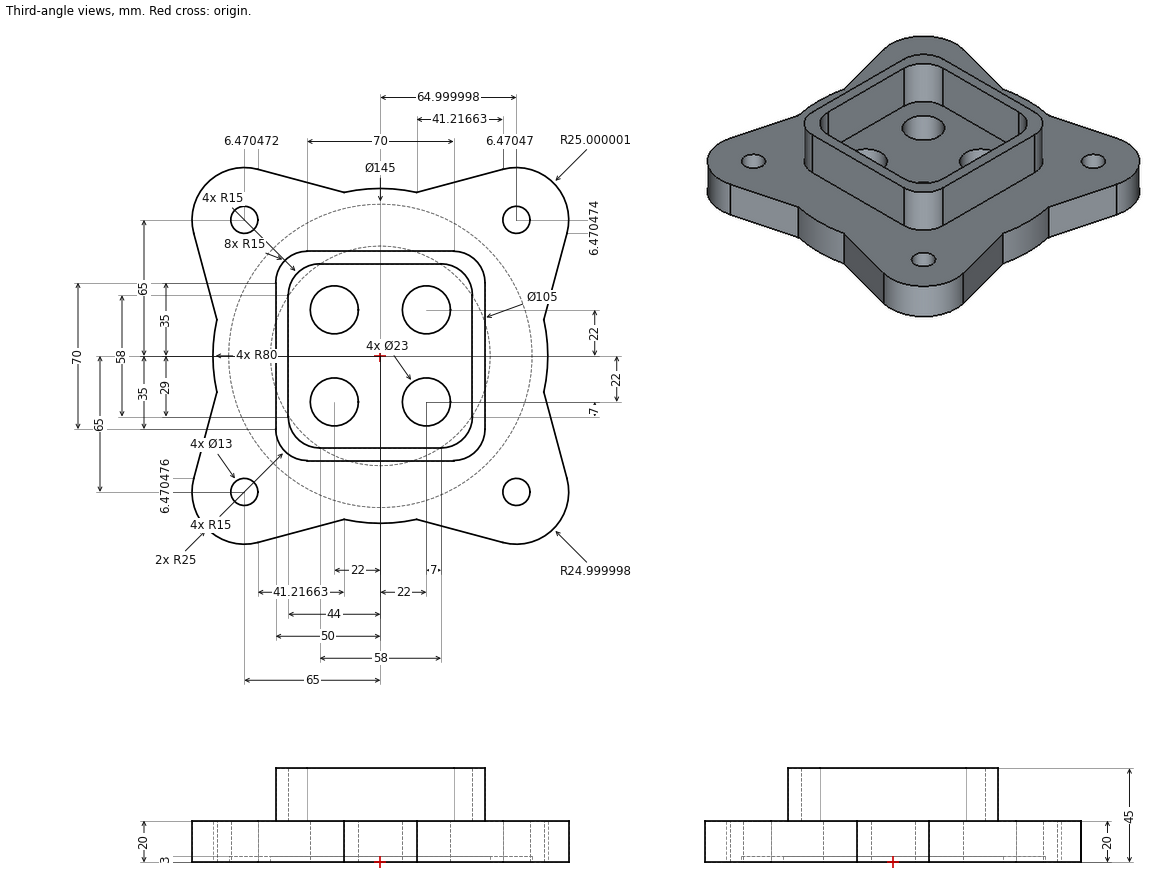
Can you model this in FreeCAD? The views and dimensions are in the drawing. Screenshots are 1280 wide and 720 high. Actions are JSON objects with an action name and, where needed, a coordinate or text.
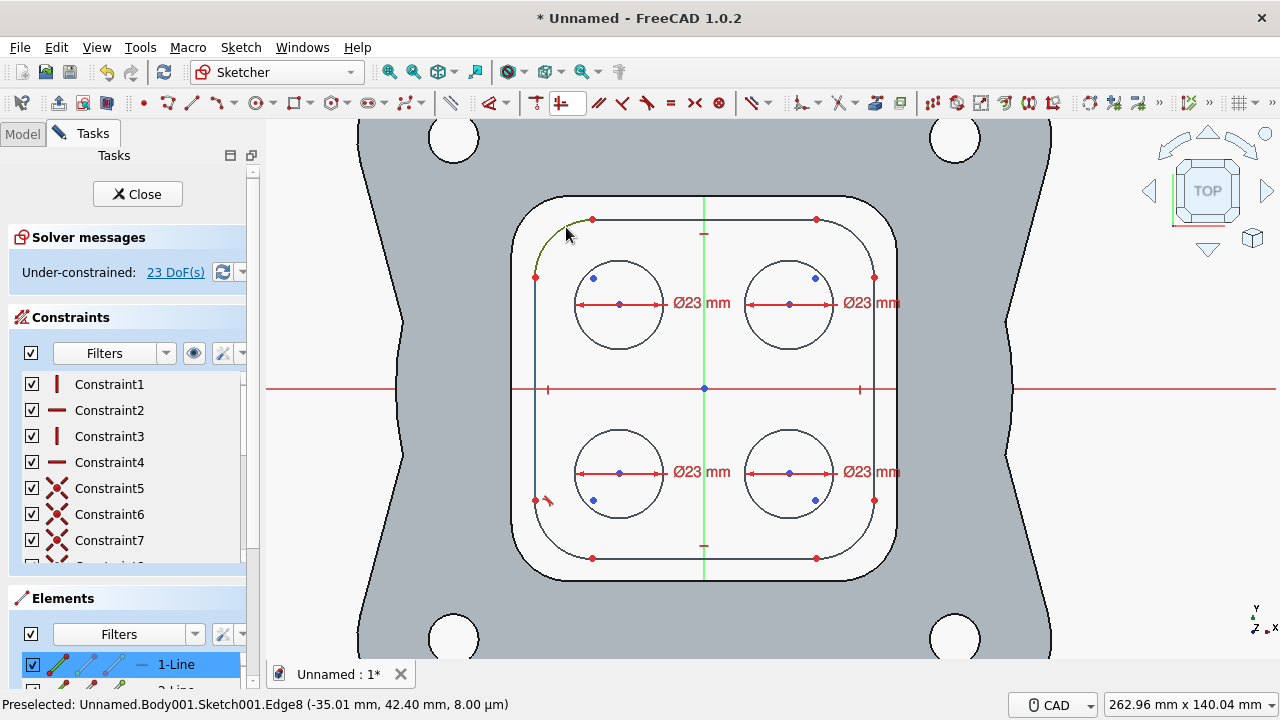
{"action": "left_click", "coordinate": [648, 104]}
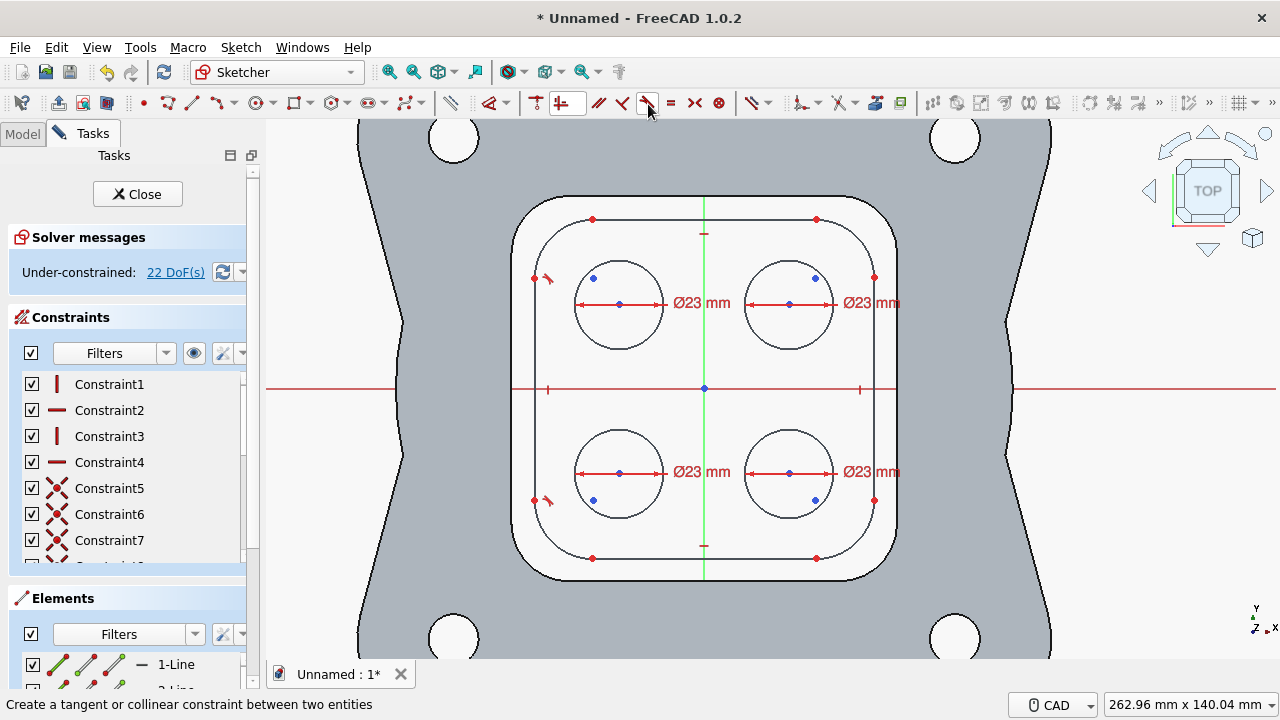
{"action": "left_click", "coordinate": [659, 559]}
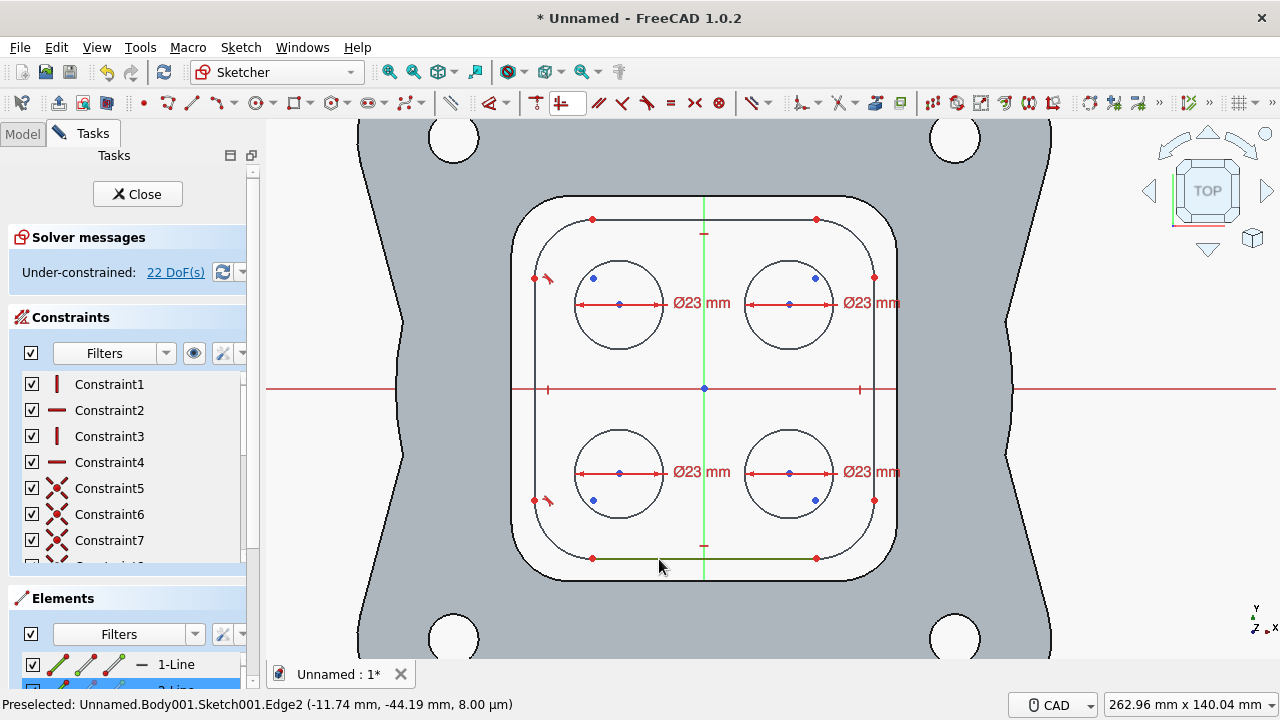
{"action": "left_click", "coordinate": [541, 527]}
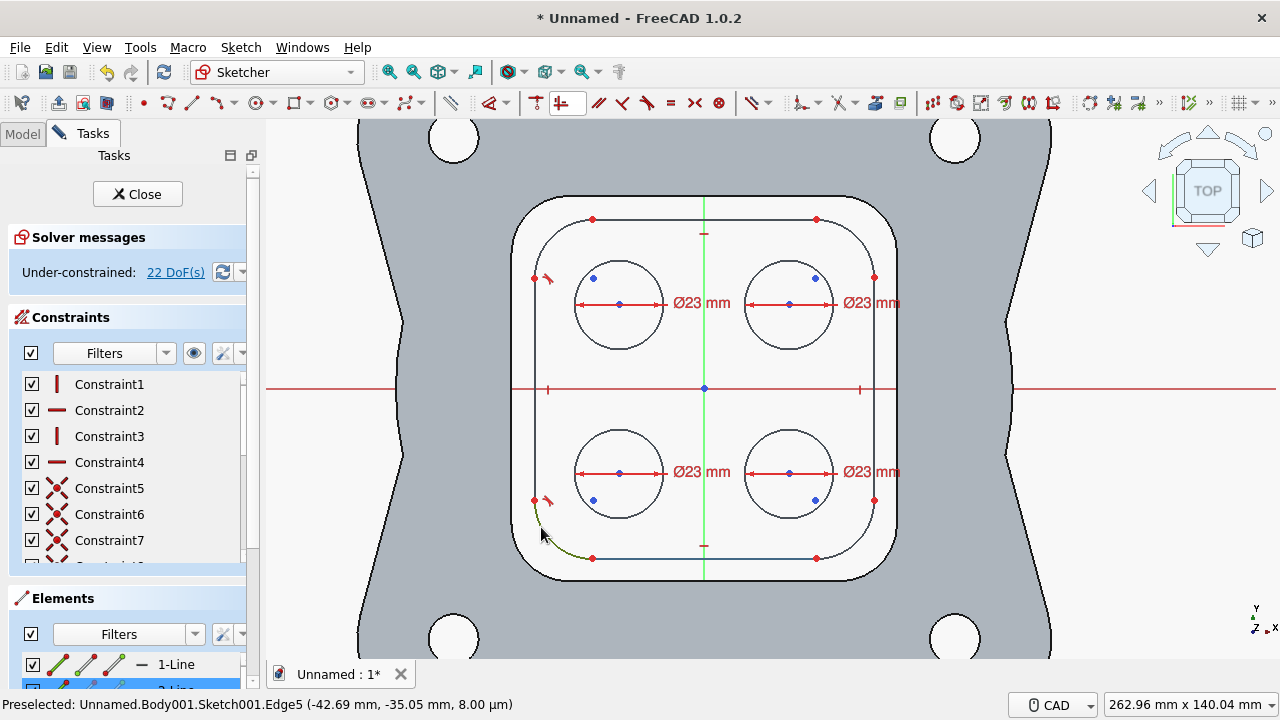
{"action": "left_click", "coordinate": [648, 104]}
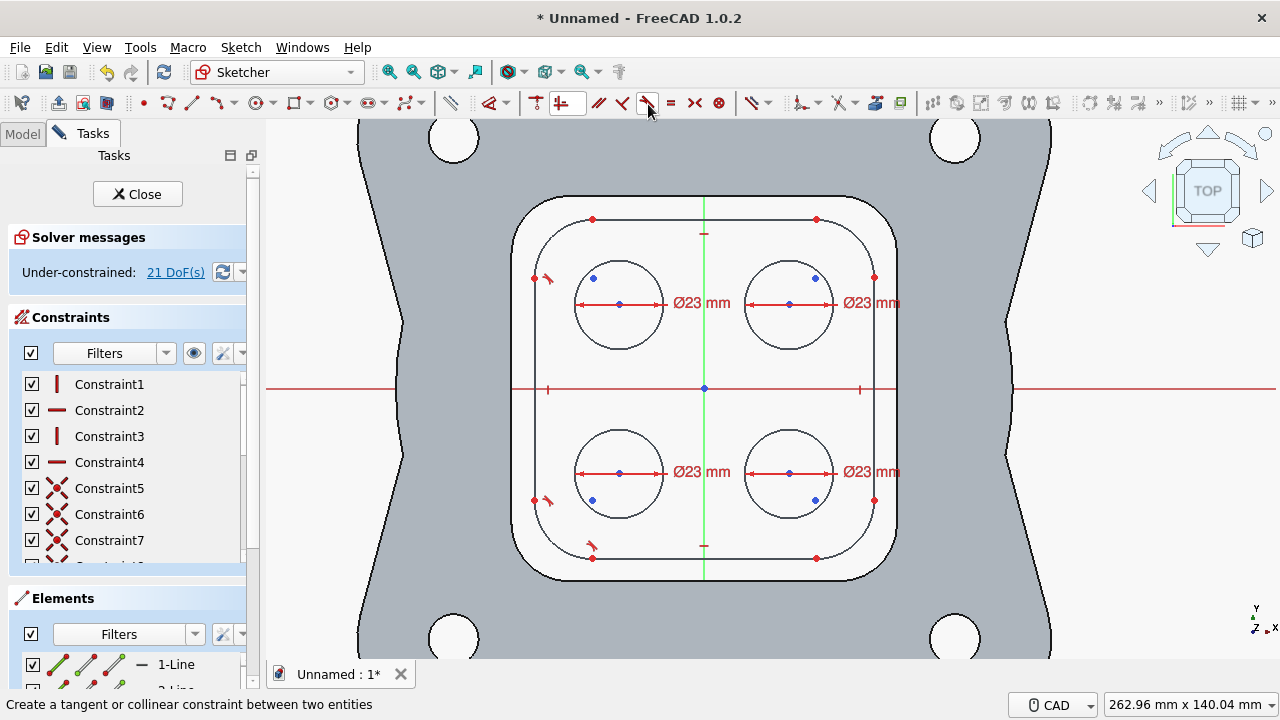
{"action": "left_click", "coordinate": [660, 559]}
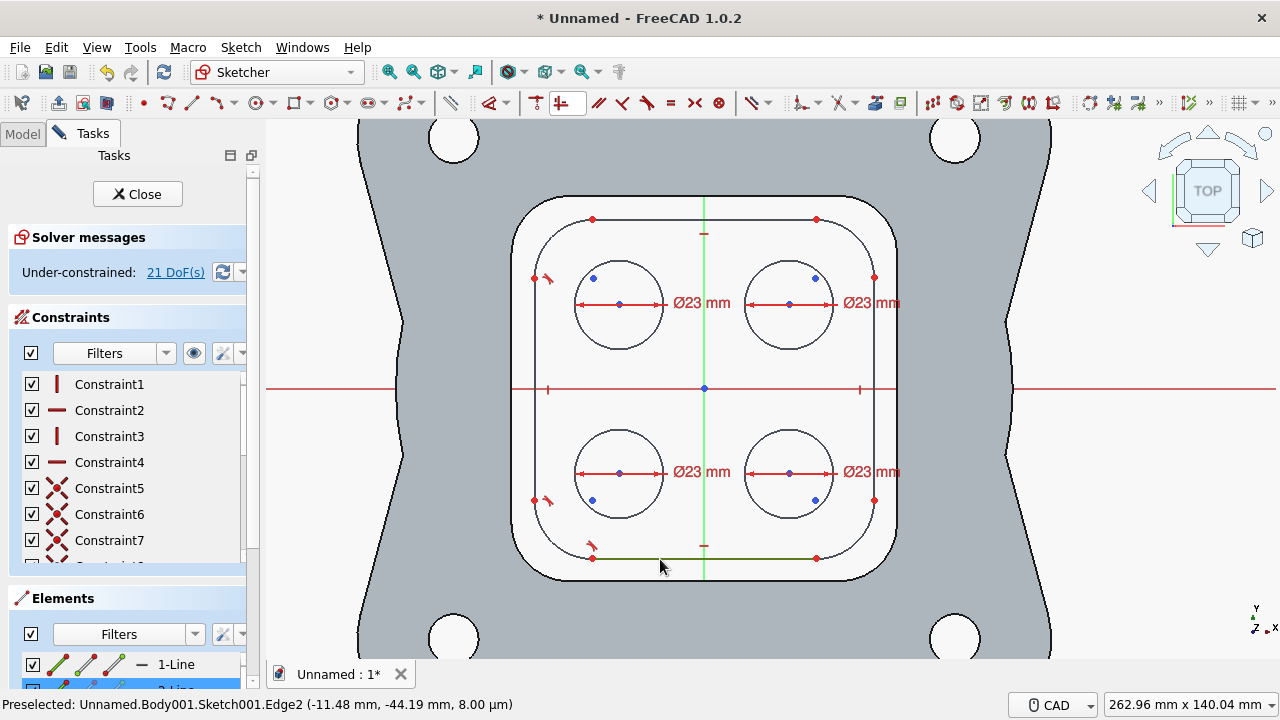
{"action": "left_click", "coordinate": [842, 553]}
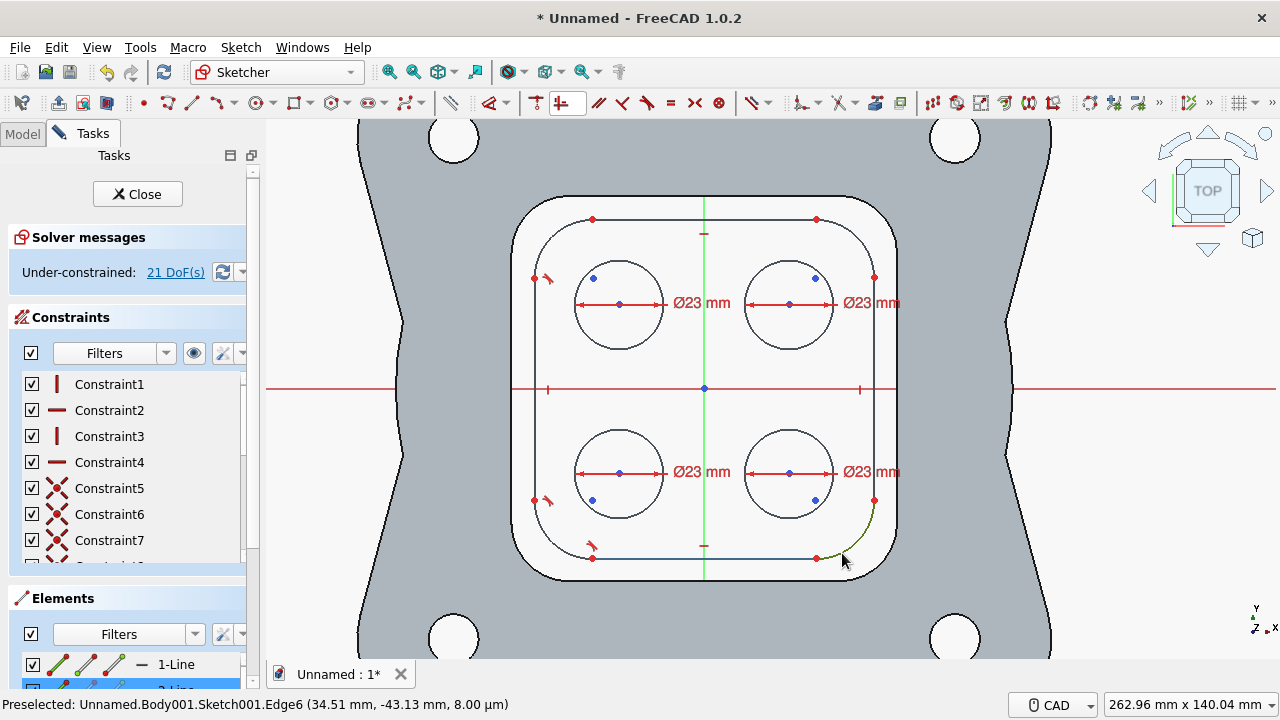
{"action": "left_click", "coordinate": [648, 104]}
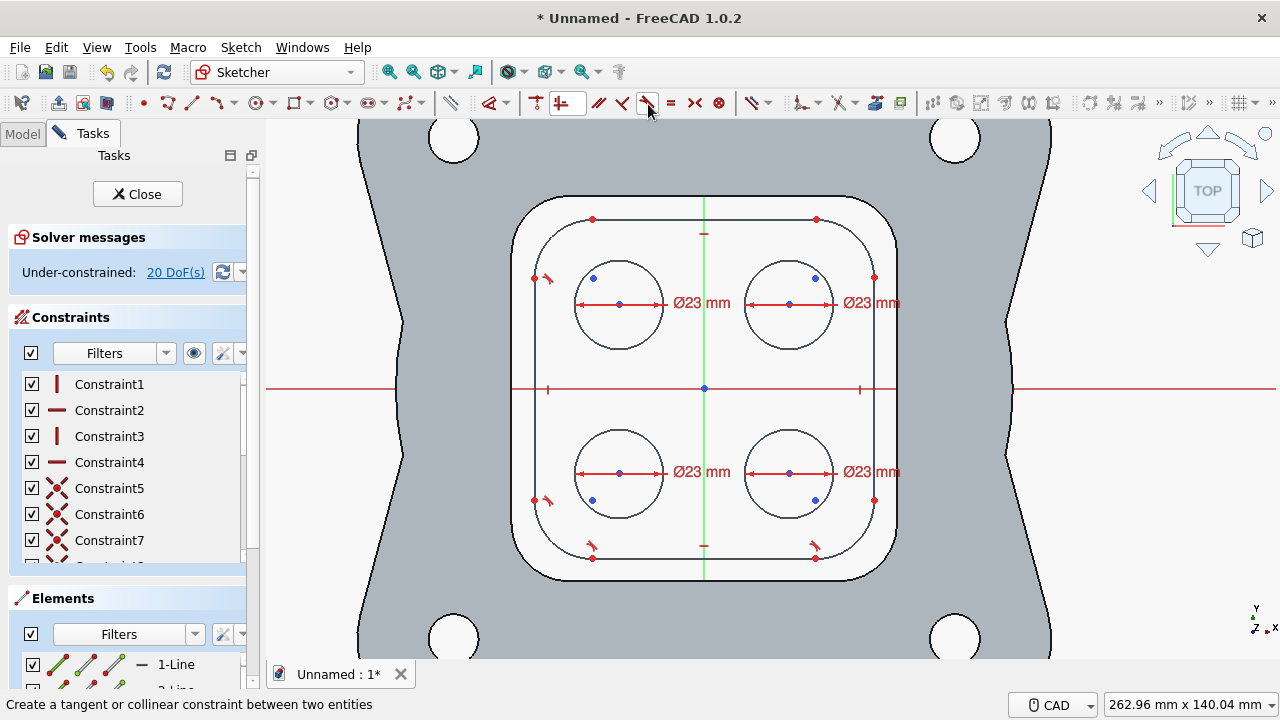
{"action": "left_click", "coordinate": [874, 434]}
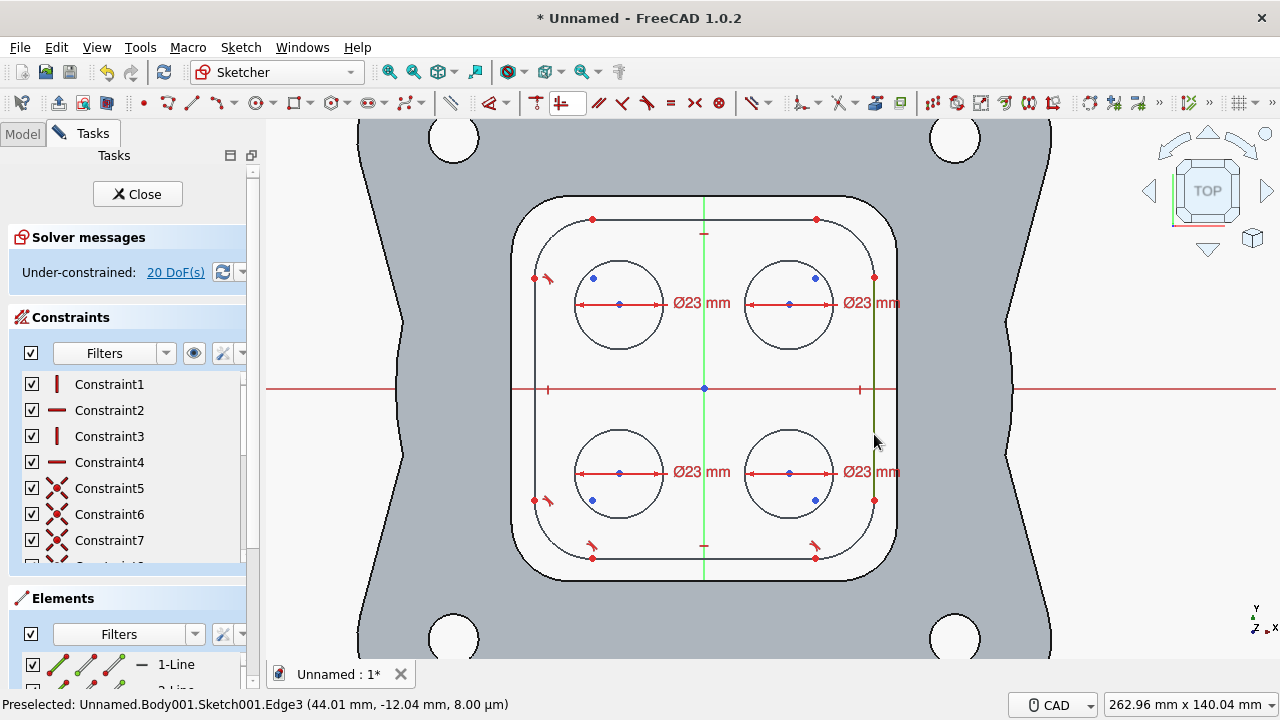
{"action": "left_click", "coordinate": [842, 553]}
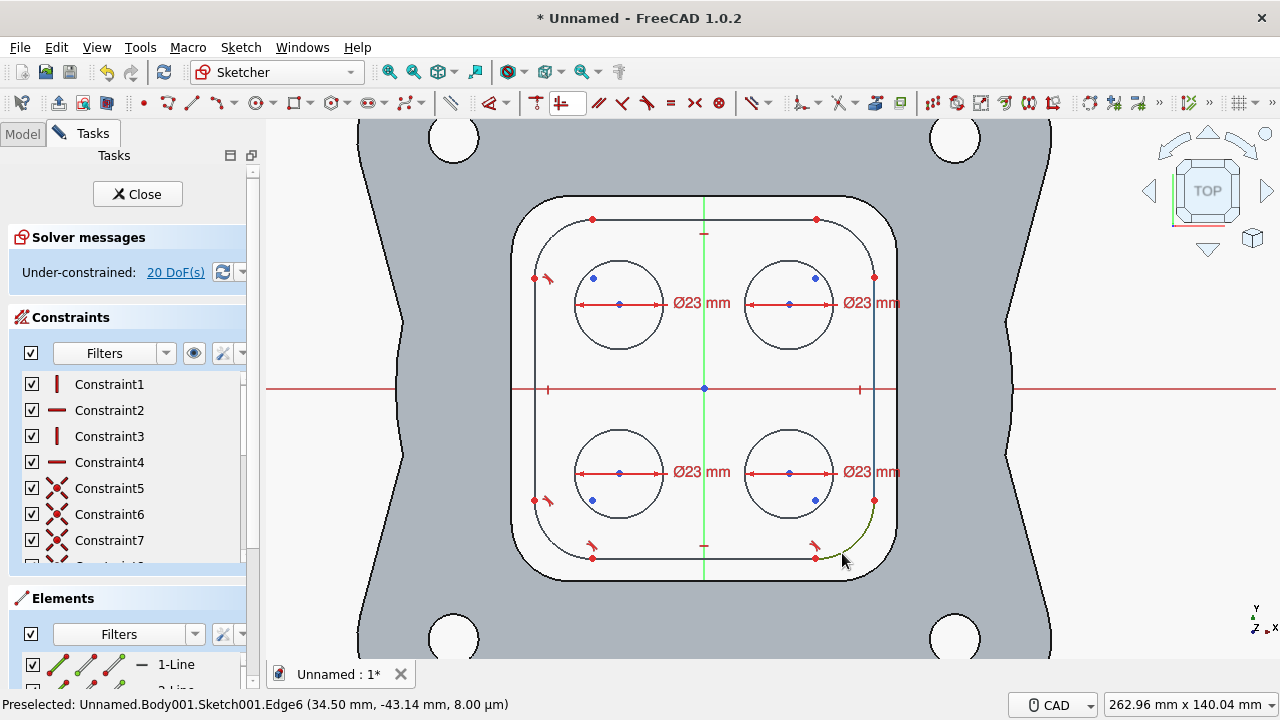
{"action": "left_click", "coordinate": [648, 104]}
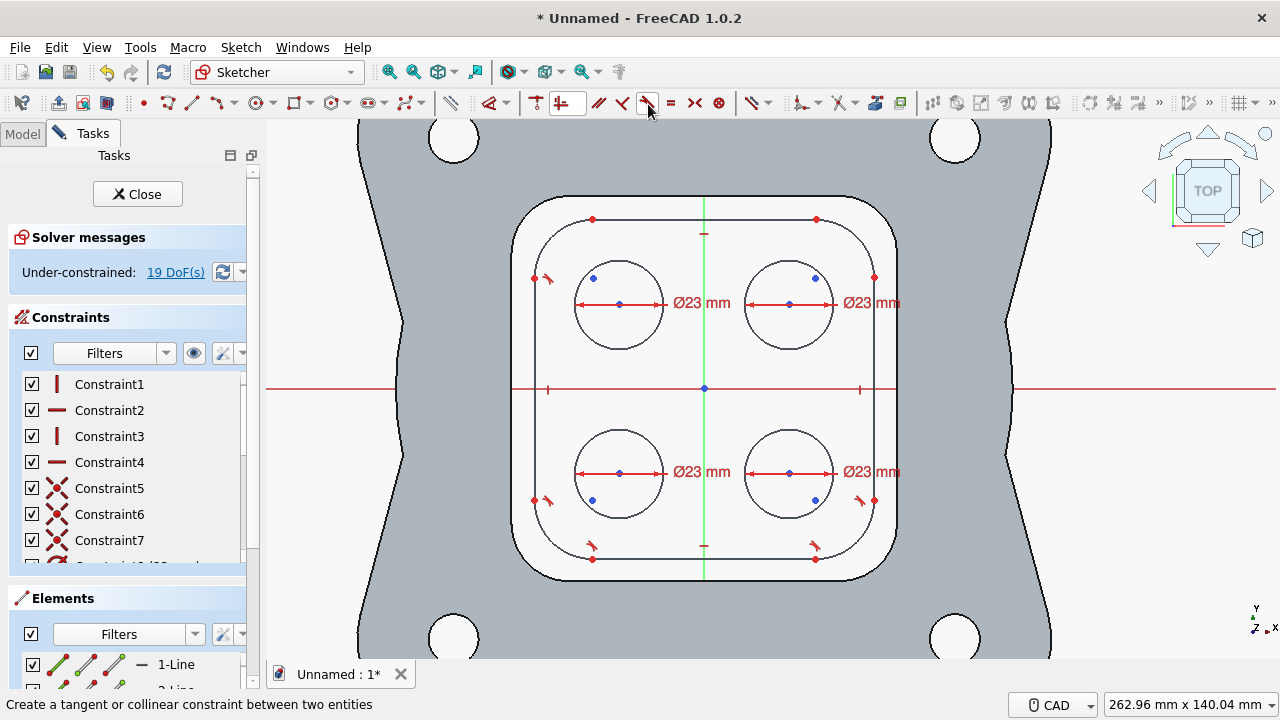
{"action": "left_click", "coordinate": [874, 434]}